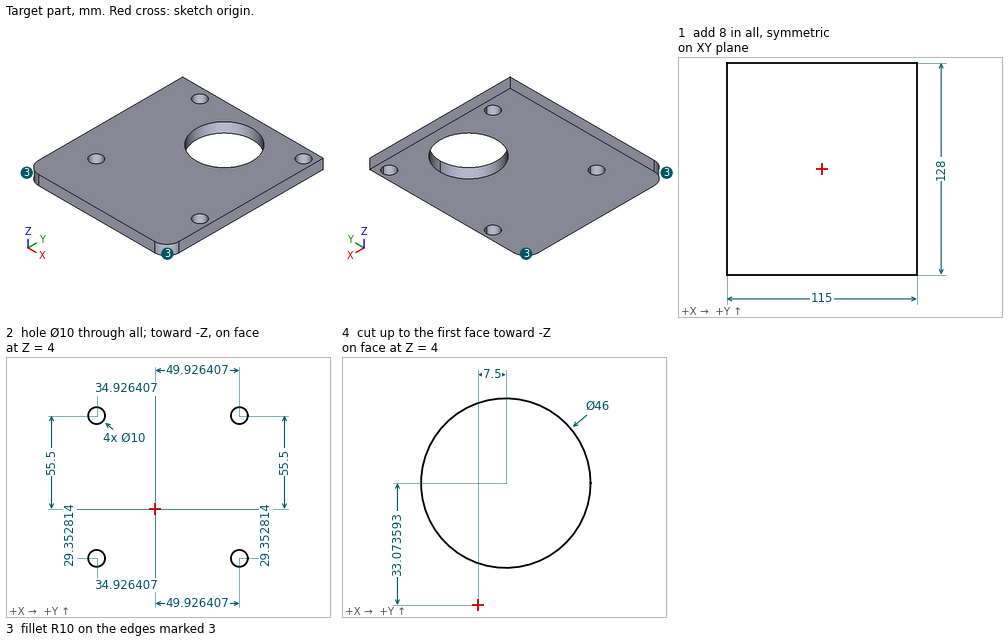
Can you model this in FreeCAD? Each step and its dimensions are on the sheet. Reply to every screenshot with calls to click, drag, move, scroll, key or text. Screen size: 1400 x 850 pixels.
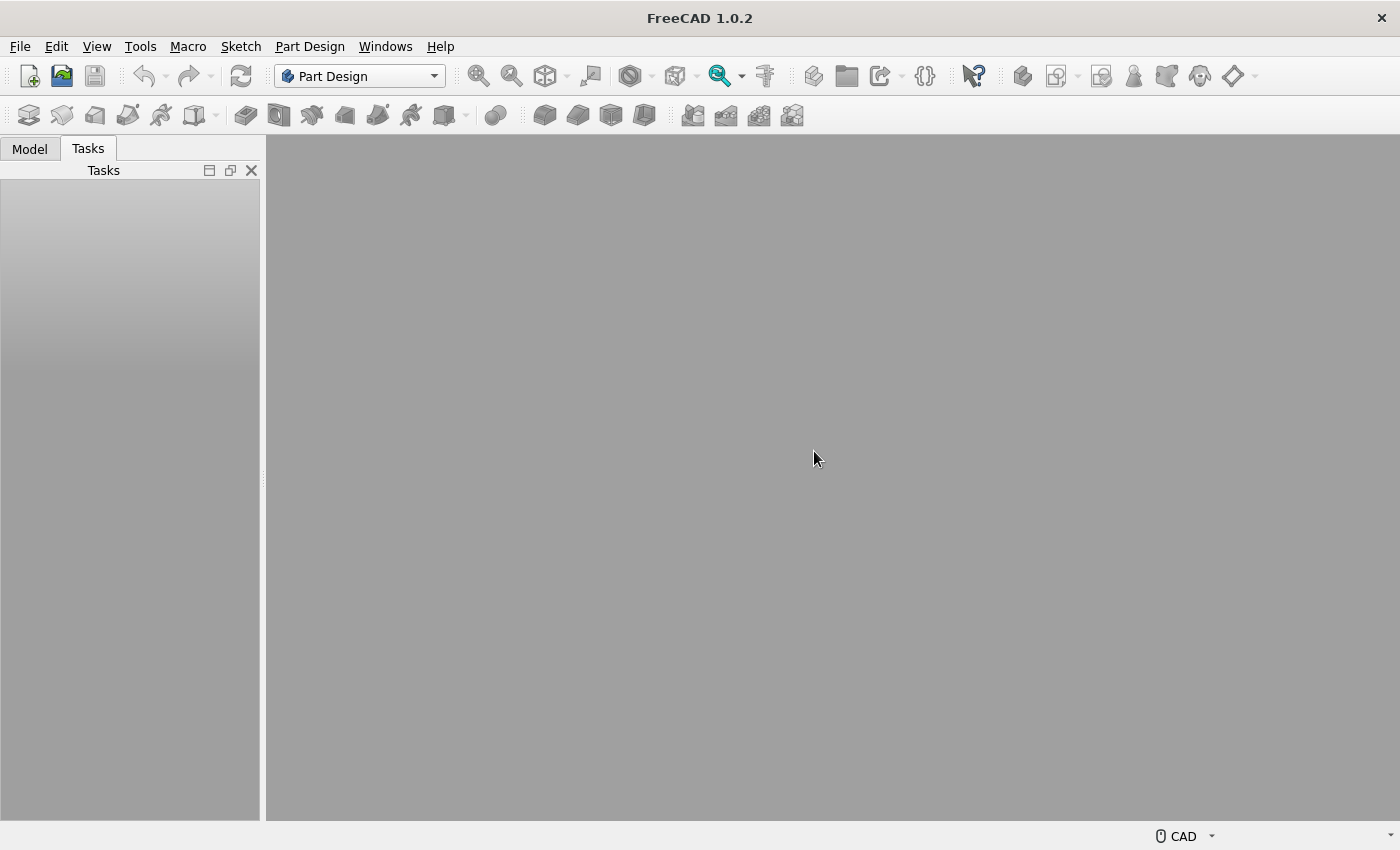
click(29, 76)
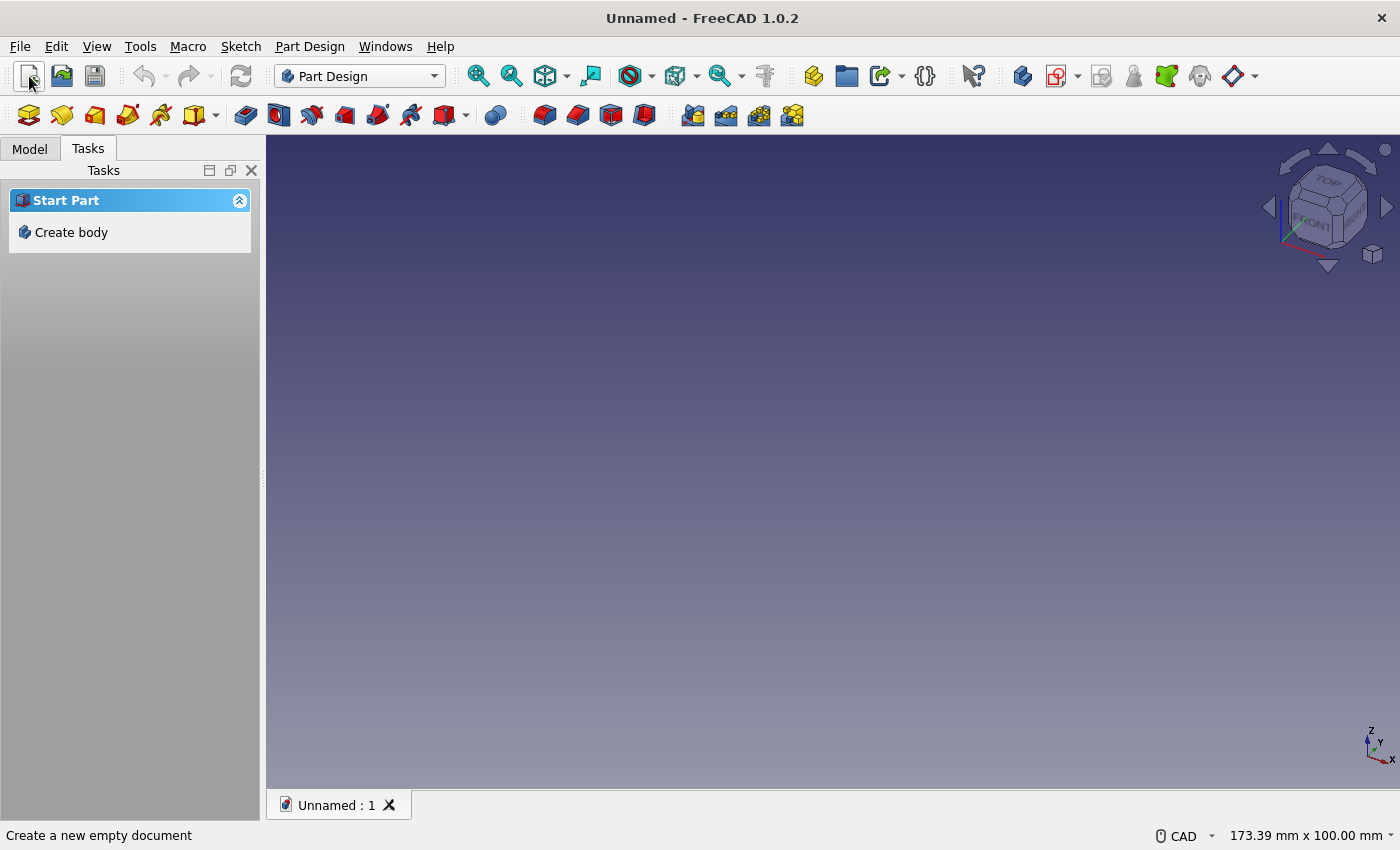
click(1056, 76)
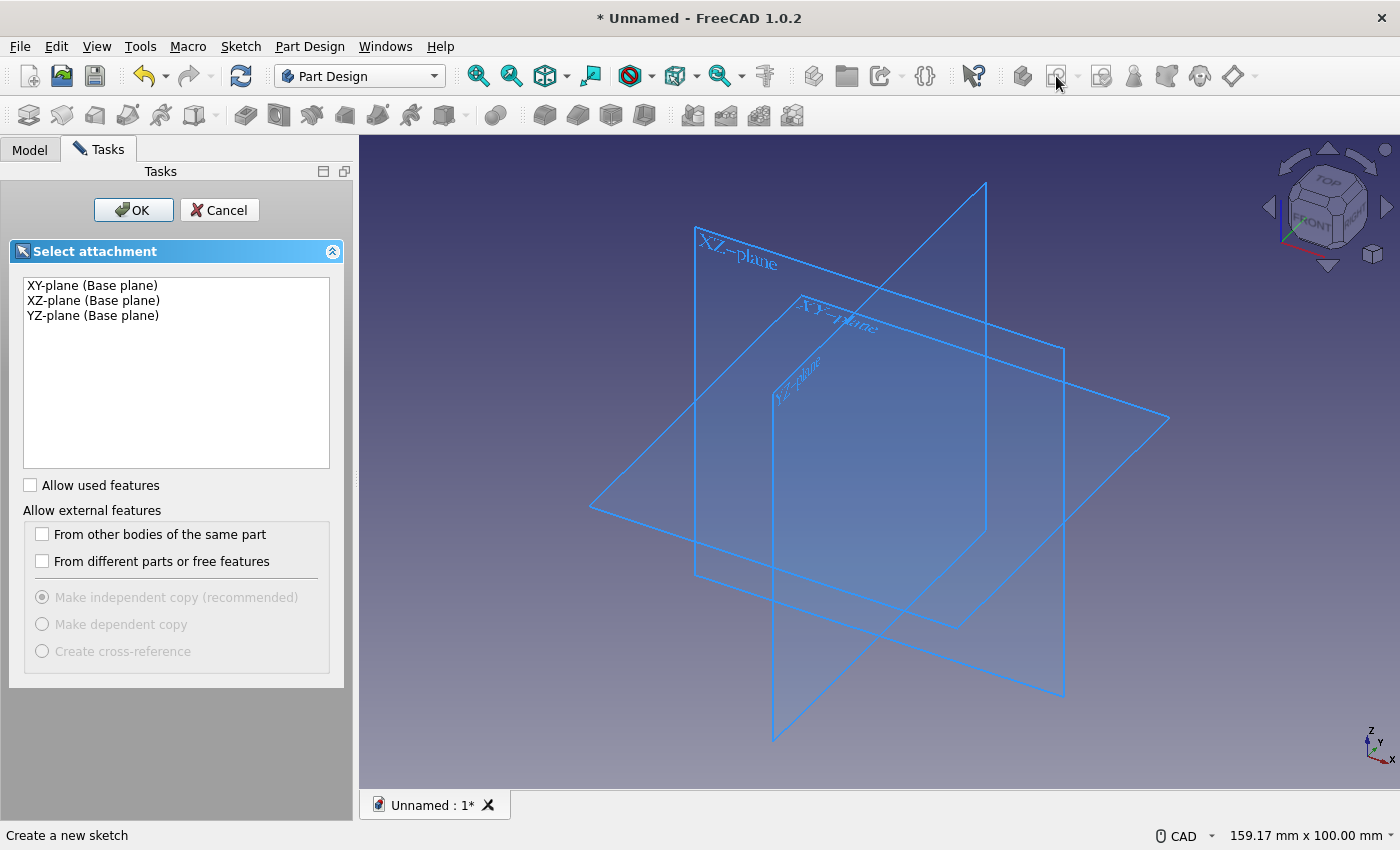
click(84, 286)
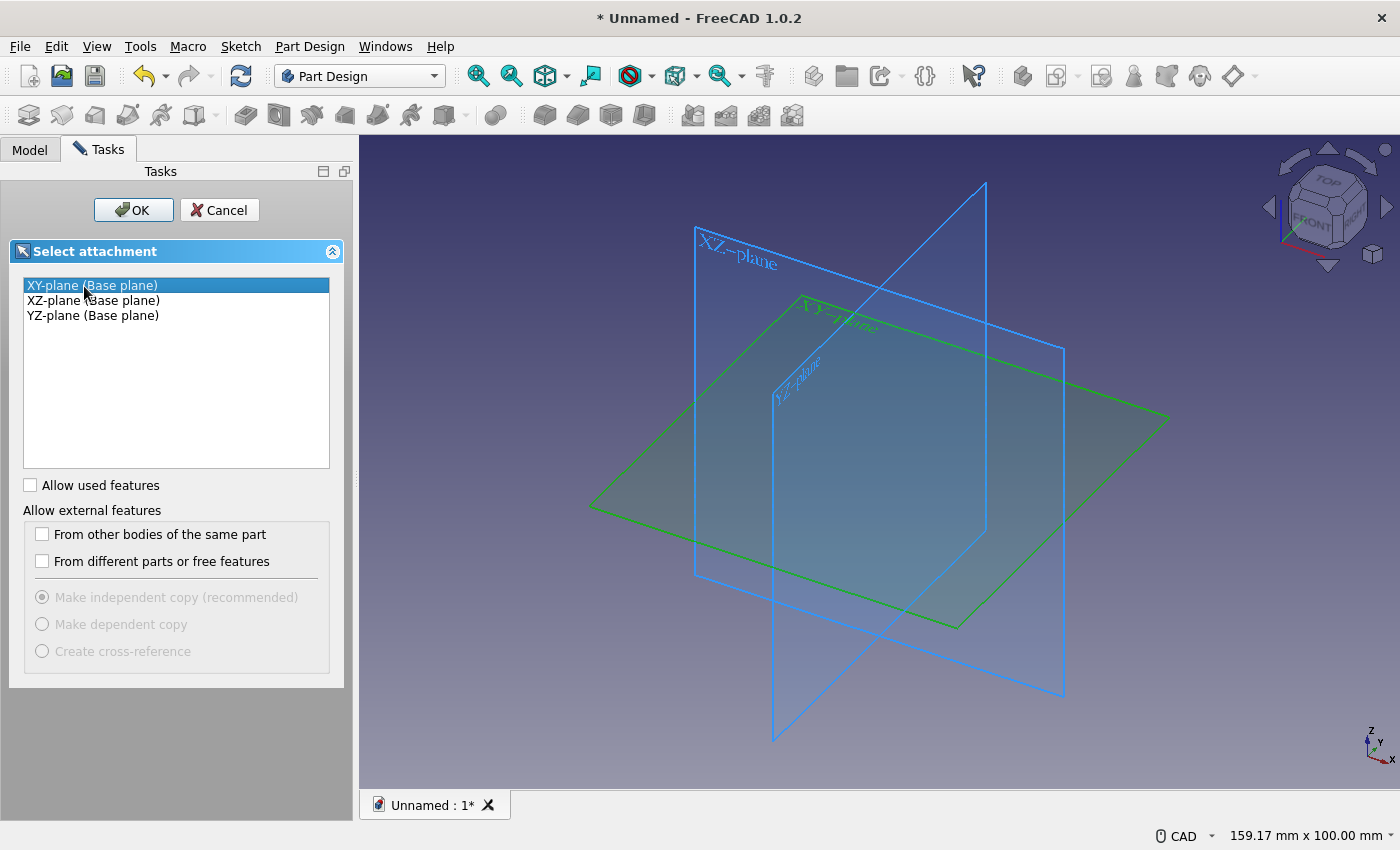
click(134, 210)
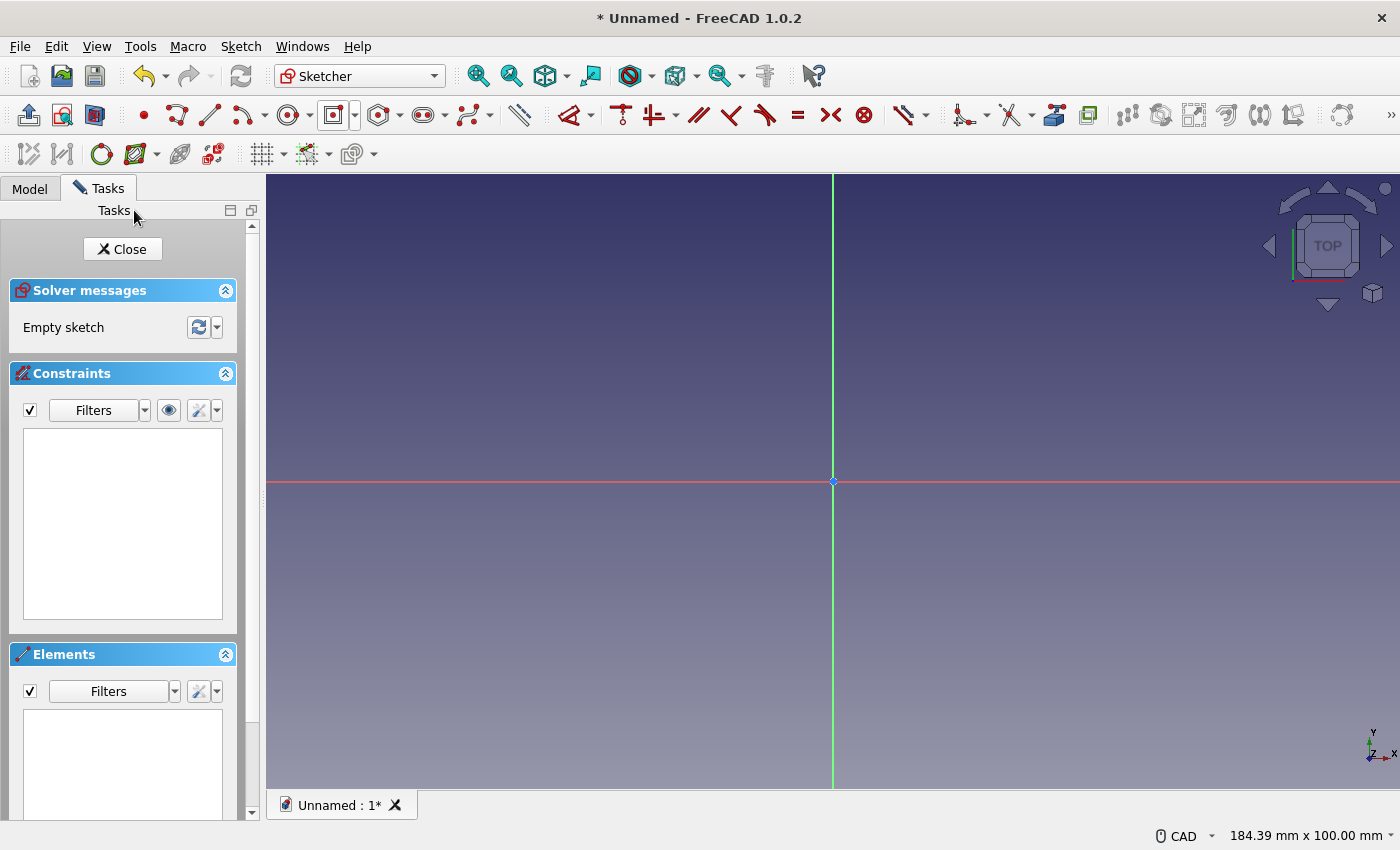
scroll(681, 482, down, 3)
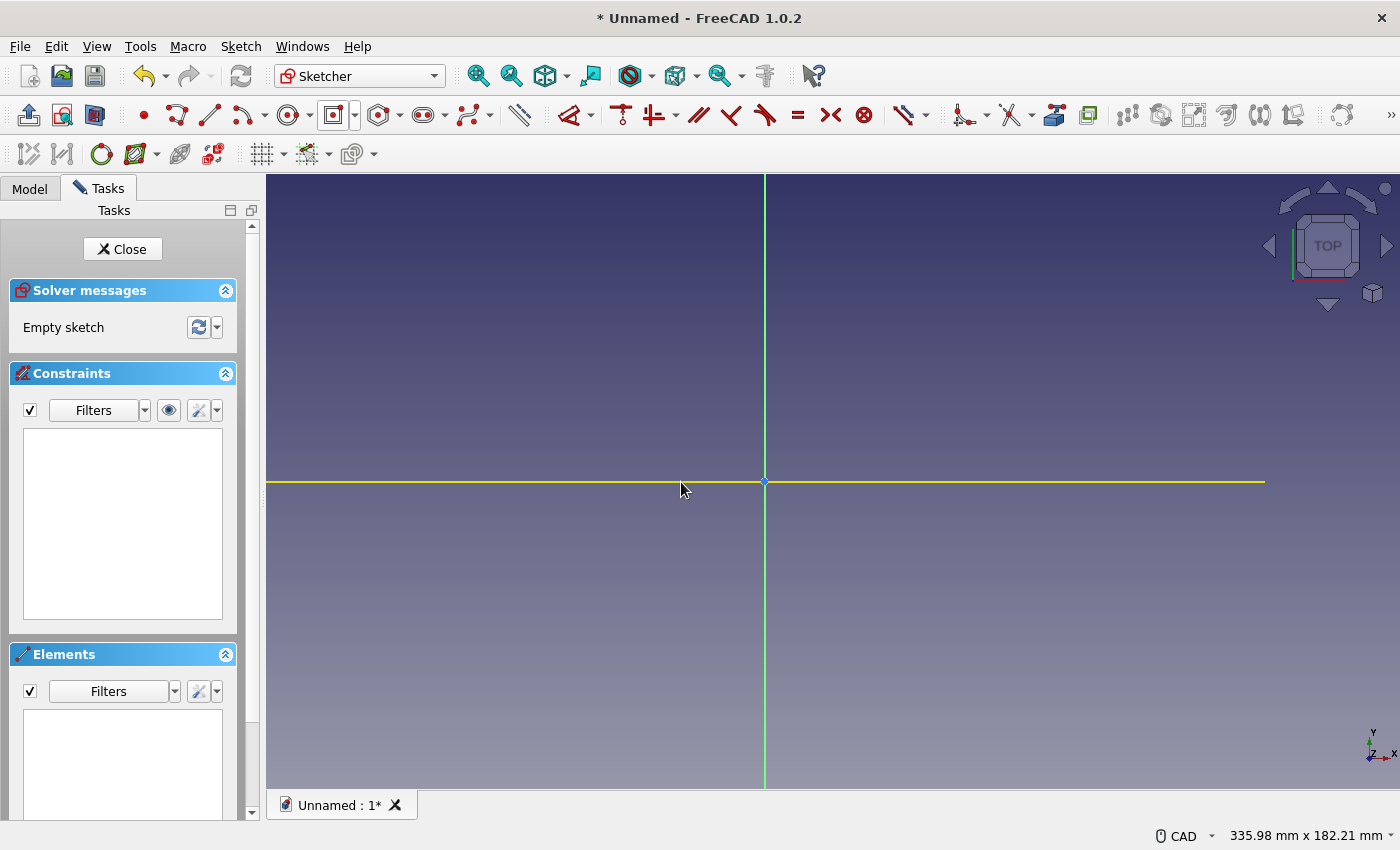
click(332, 116)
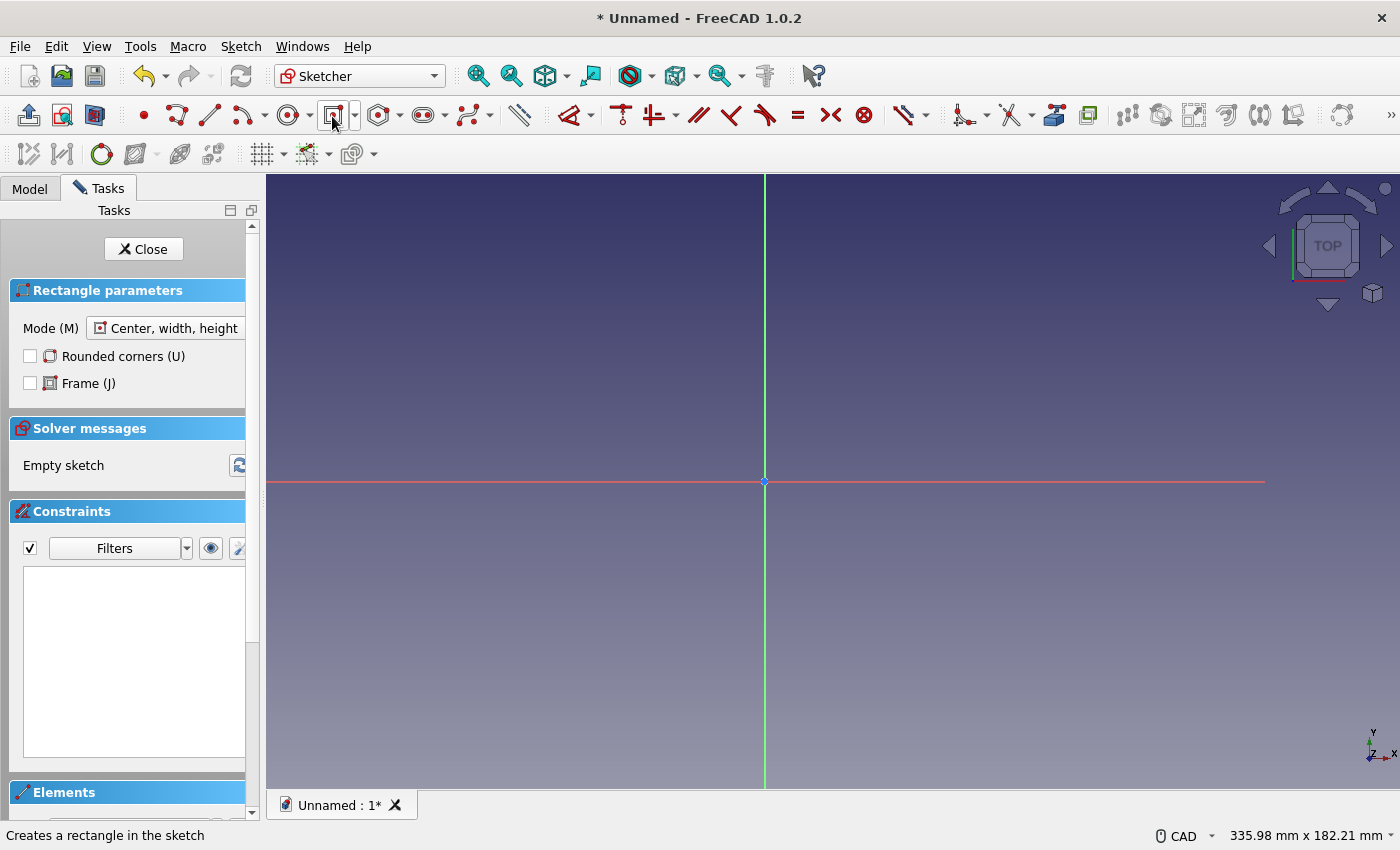
click(765, 482)
move(959, 266)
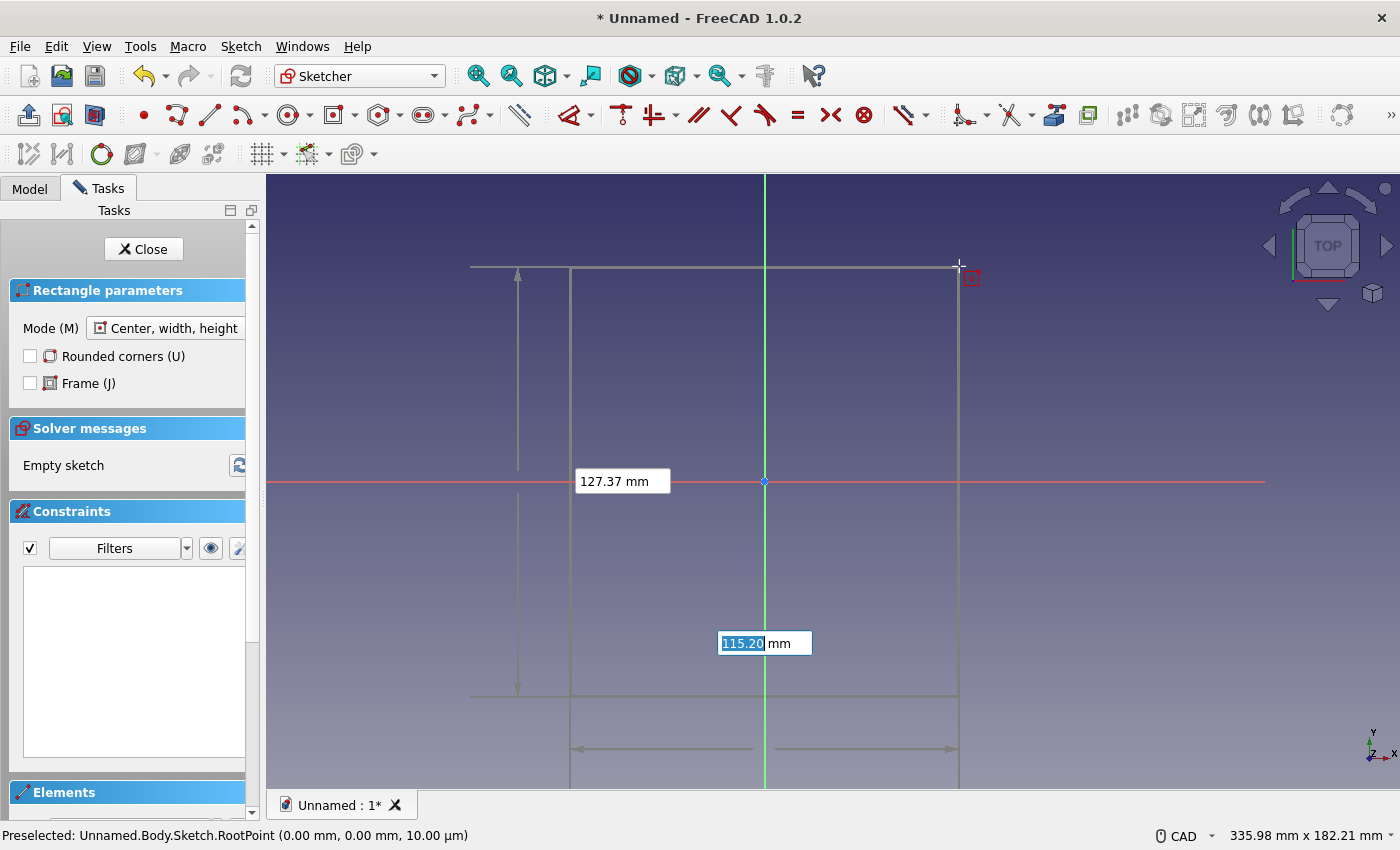
text(115)
key(Tab)
text(128)
key(Return)
key(Escape)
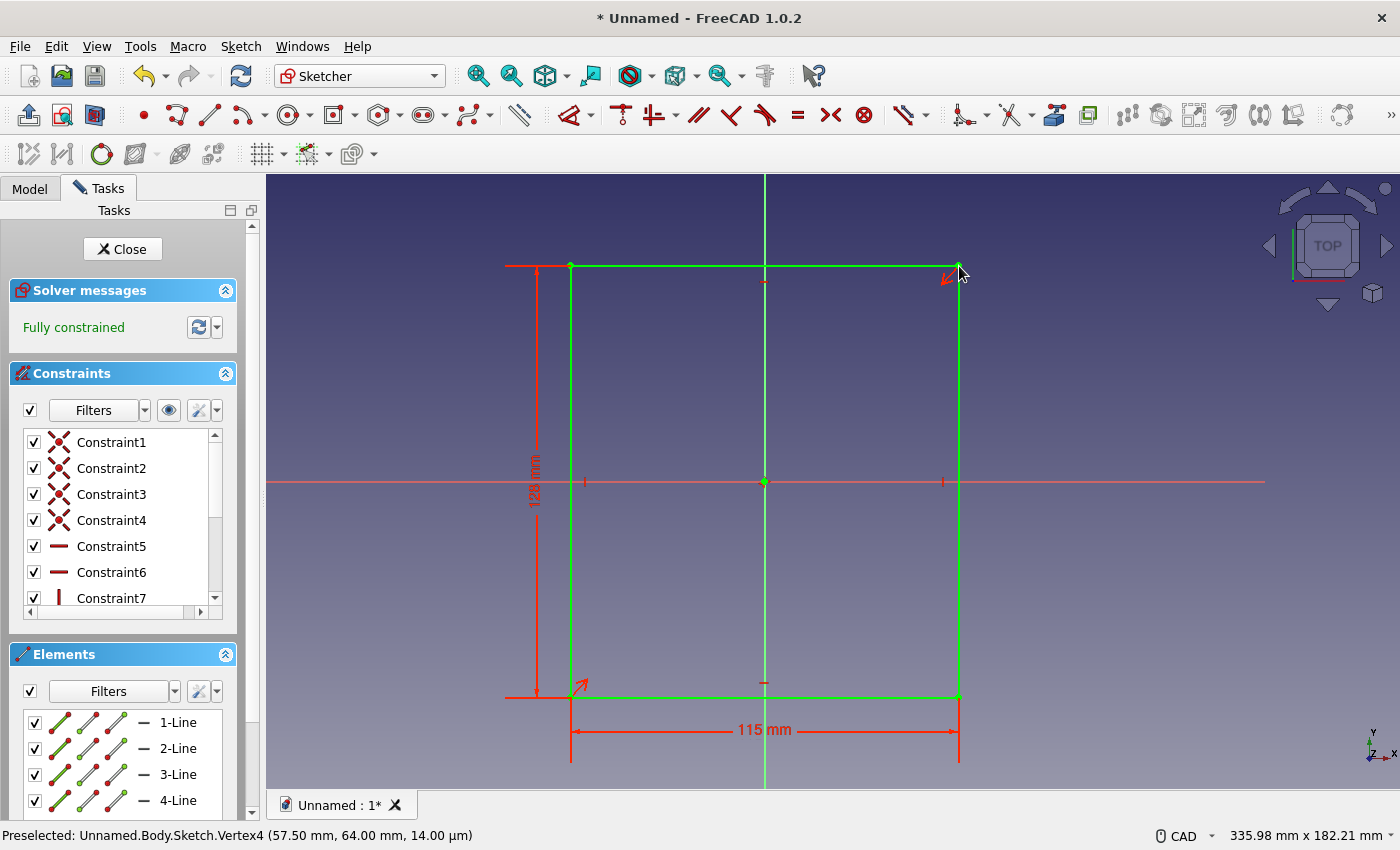
click(123, 249)